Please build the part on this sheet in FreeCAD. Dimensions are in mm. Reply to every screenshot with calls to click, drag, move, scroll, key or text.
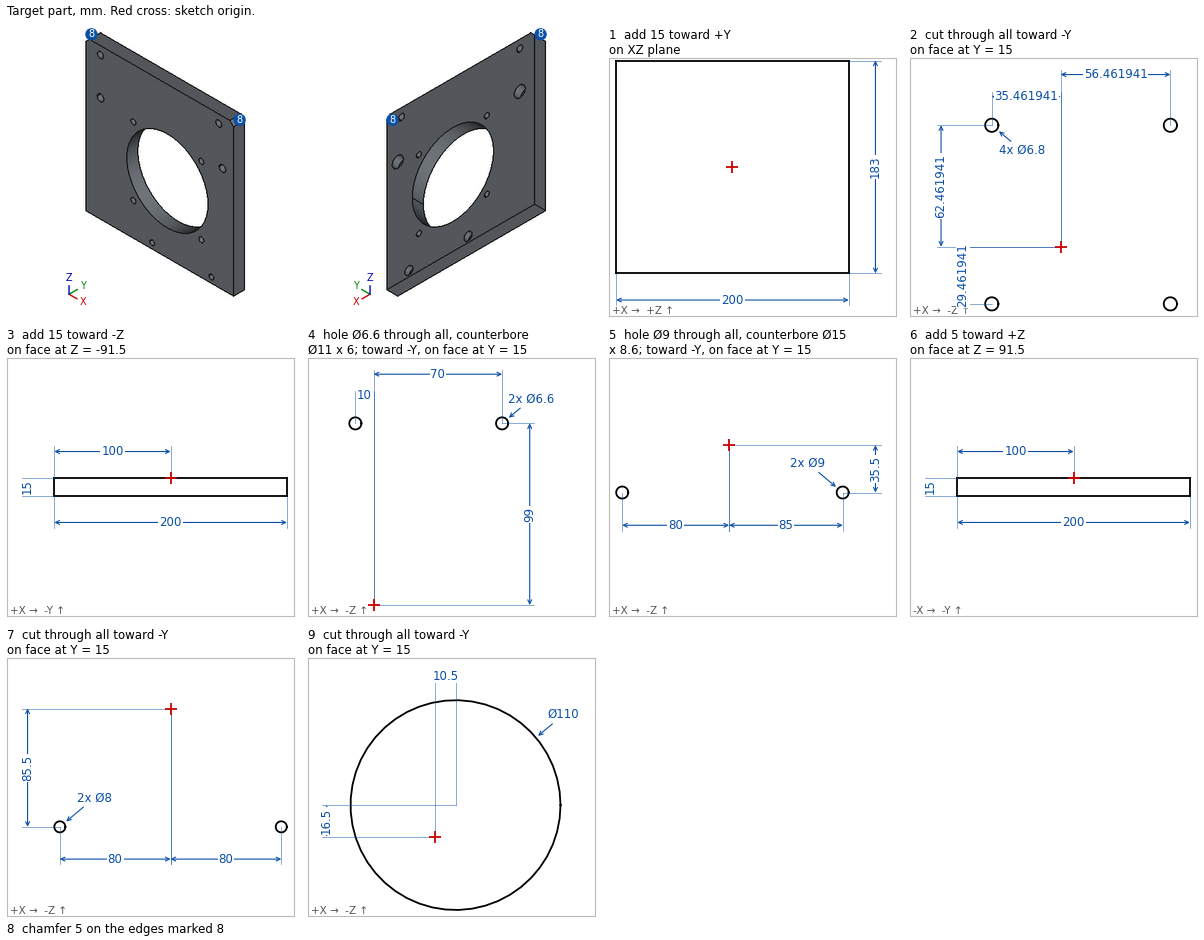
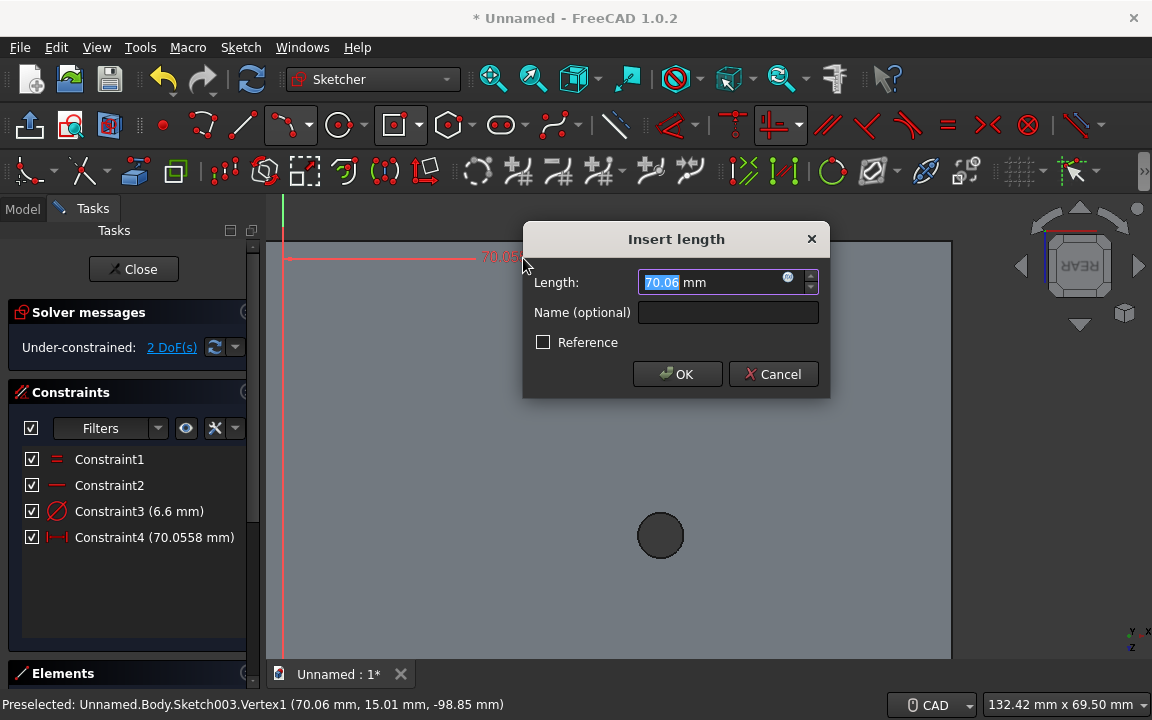
text(70)
key(Return)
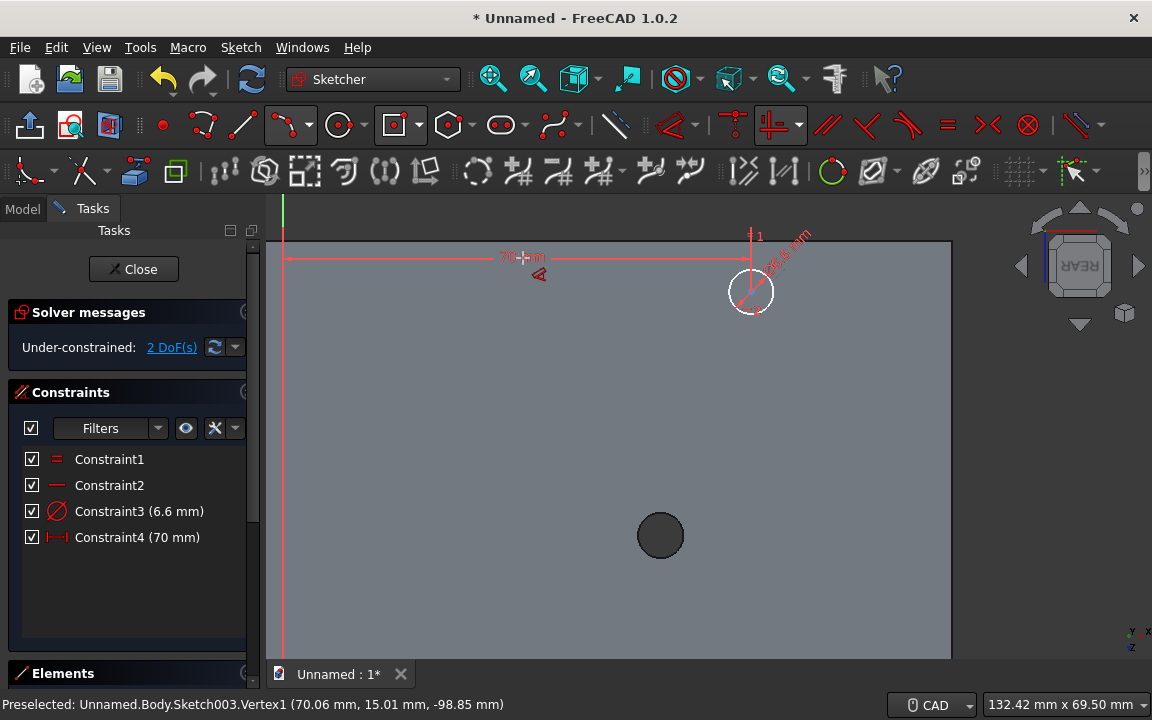
click(751, 292)
click(785, 461)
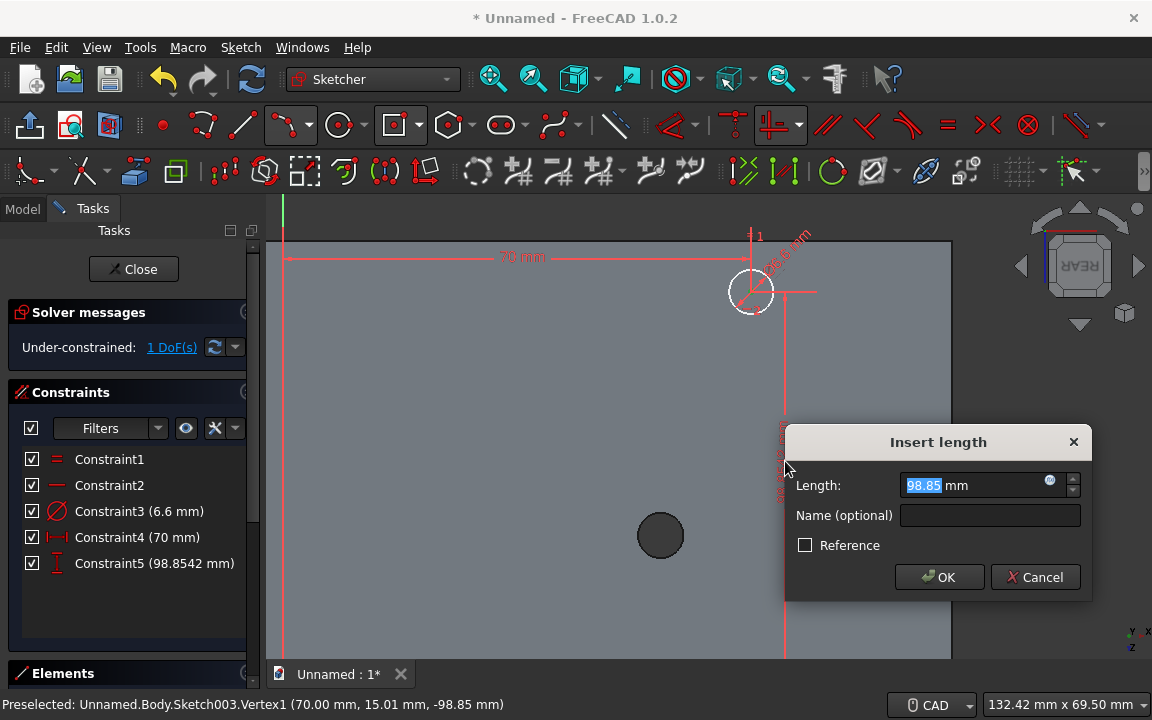
text(99)
key(Return)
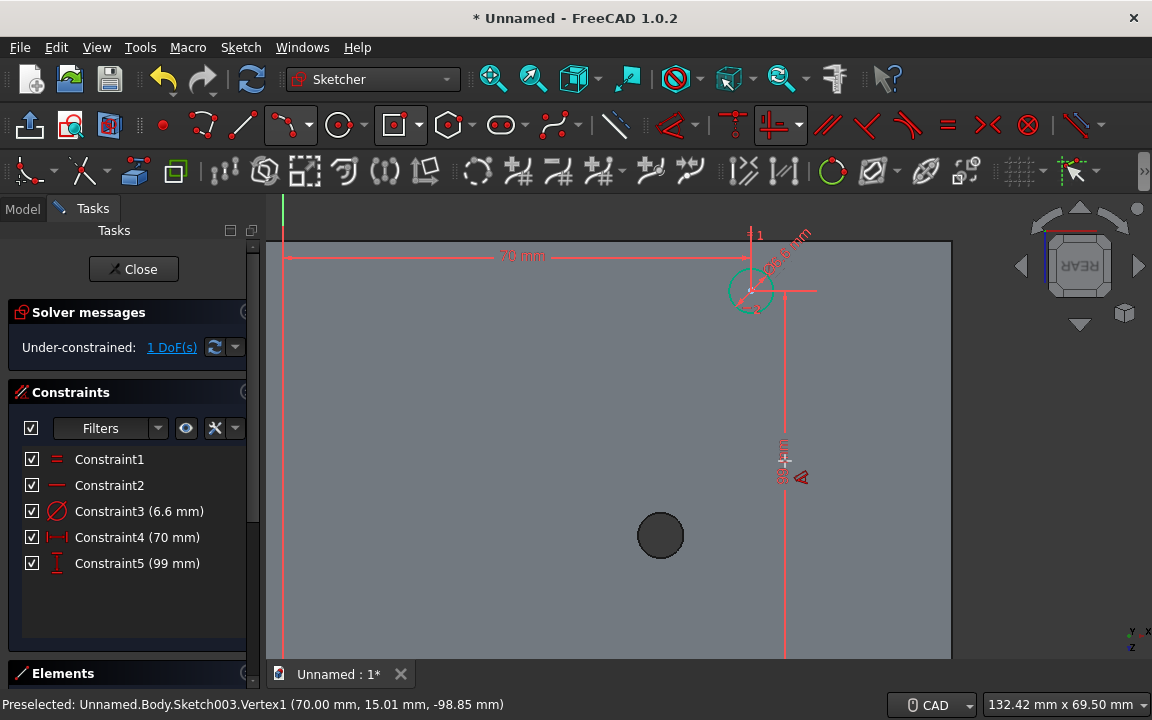
scroll(768, 276, down, 4)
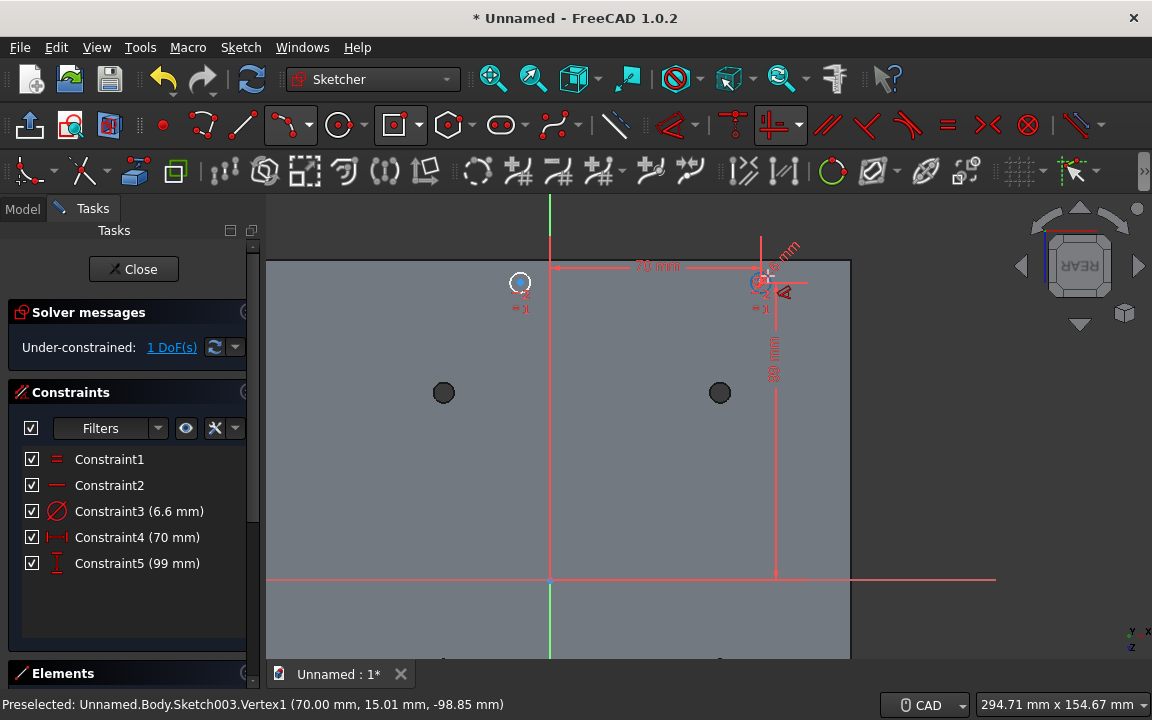
scroll(520, 283, up, 2)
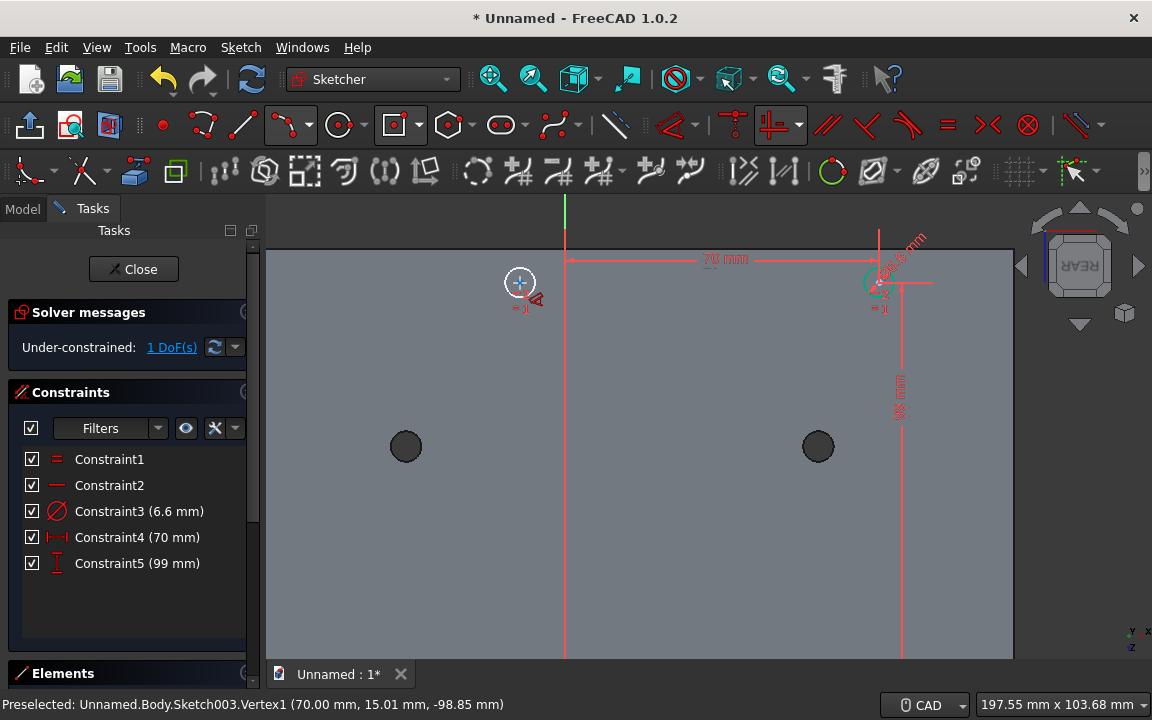
click(520, 283)
click(543, 249)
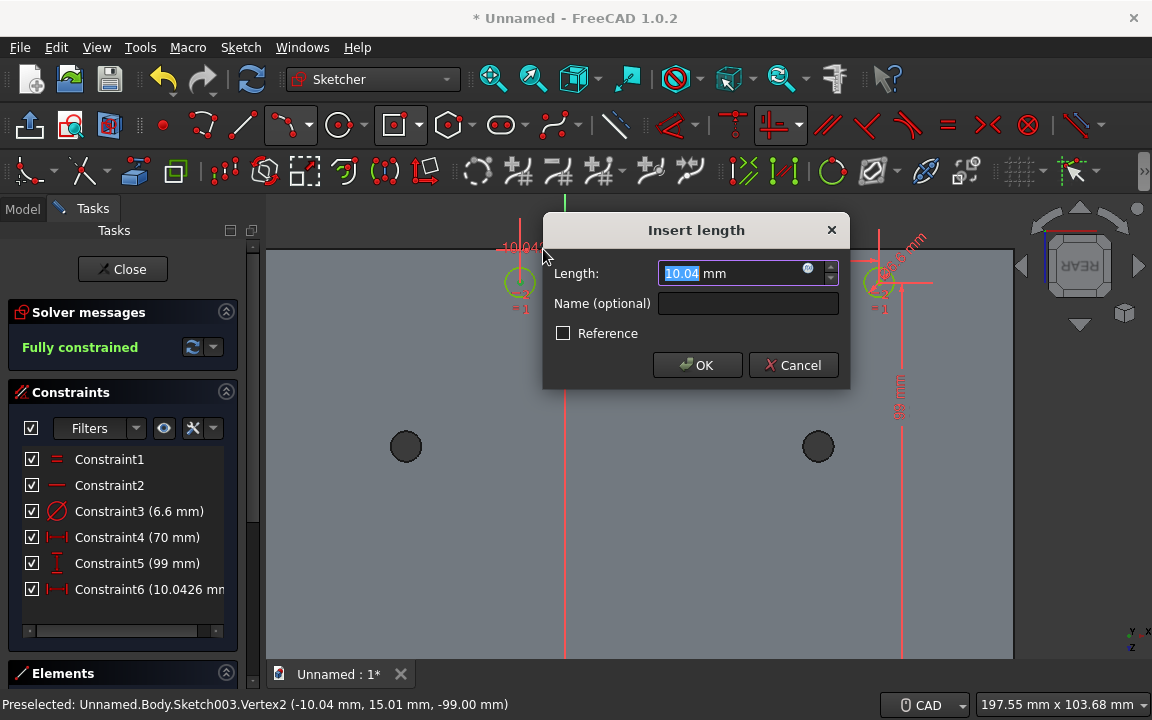
text(10)
key(Return)
key(Escape)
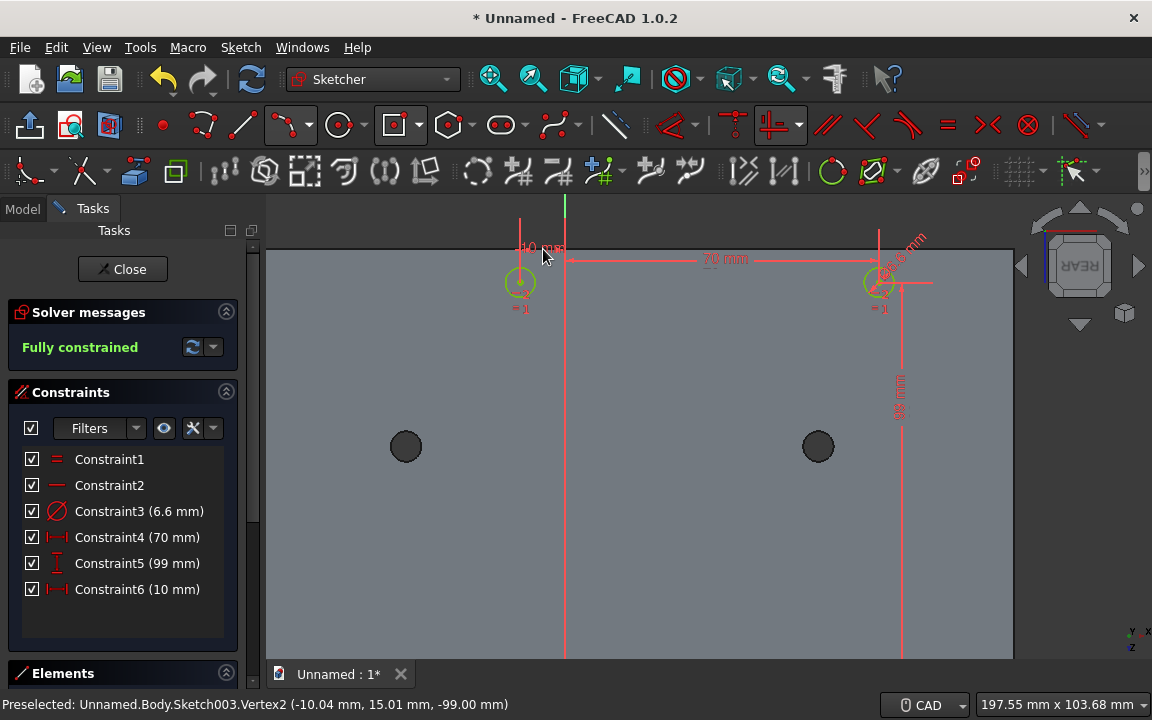
click(123, 269)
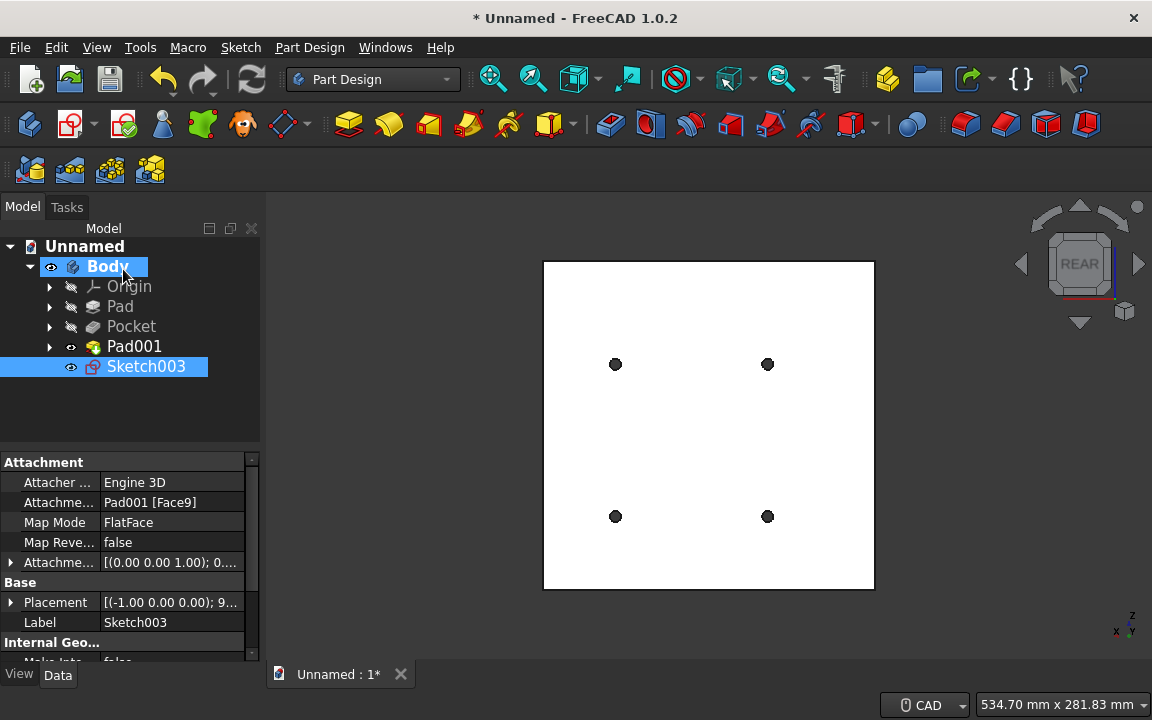
click(652, 124)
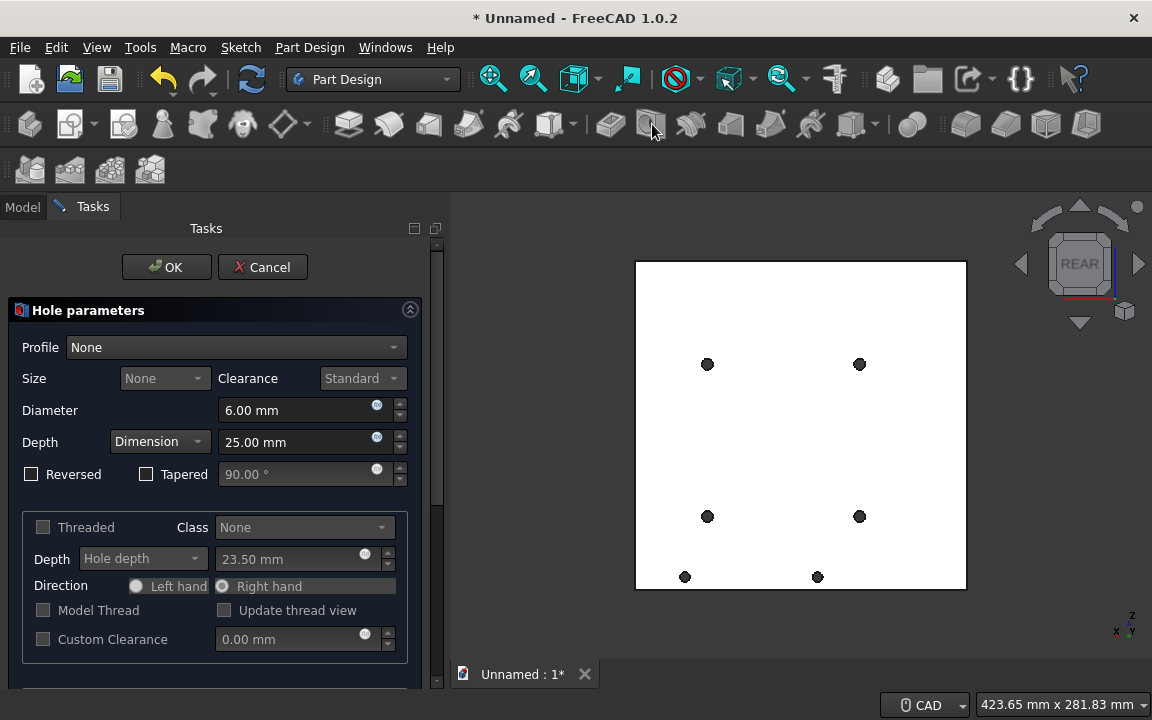
triple_click(305, 410)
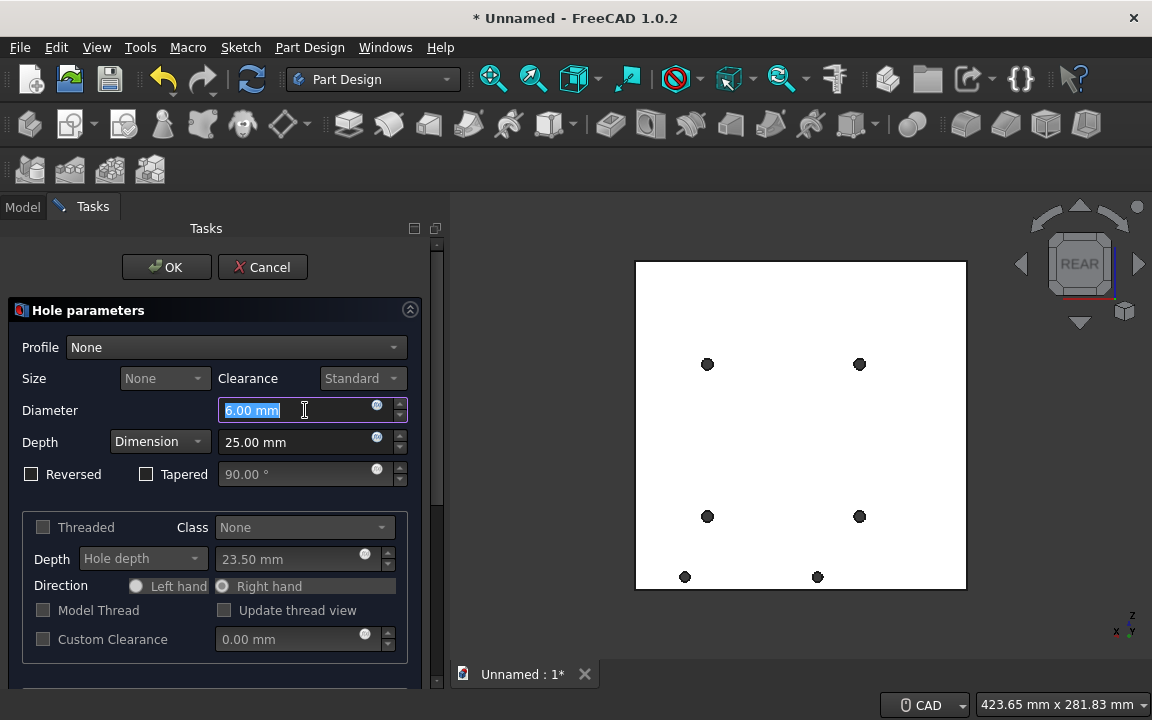
text(6.6)
key(Tab)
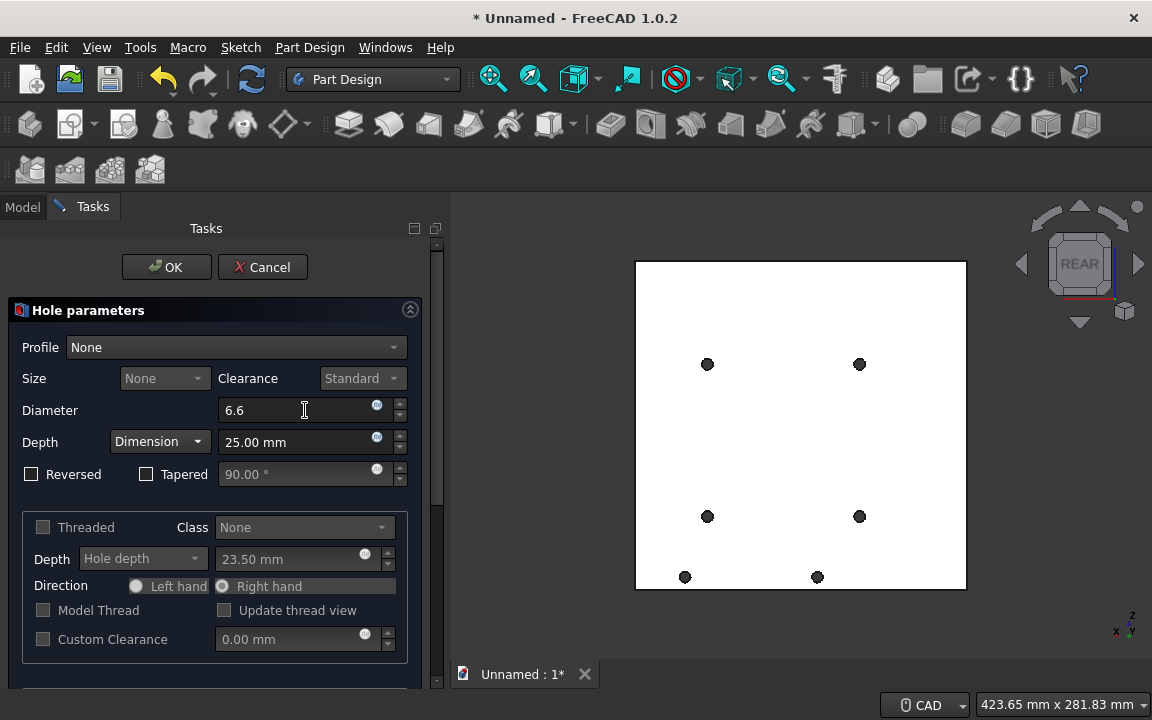
click(161, 442)